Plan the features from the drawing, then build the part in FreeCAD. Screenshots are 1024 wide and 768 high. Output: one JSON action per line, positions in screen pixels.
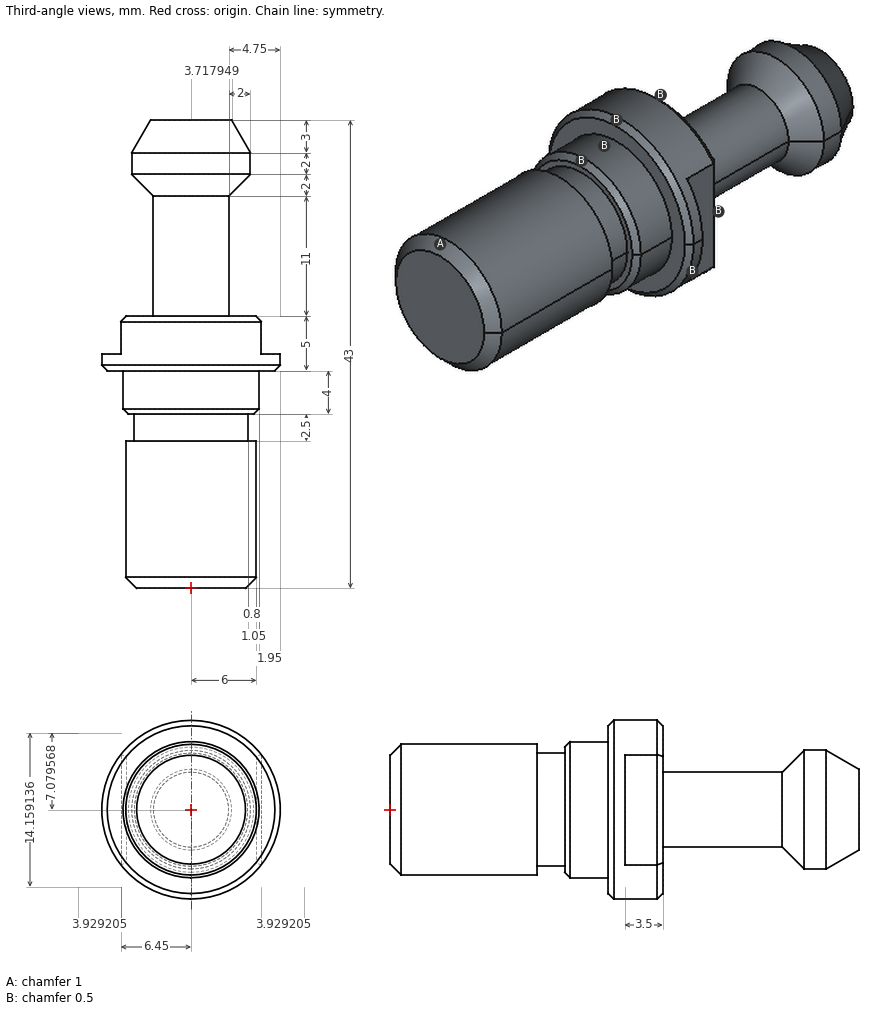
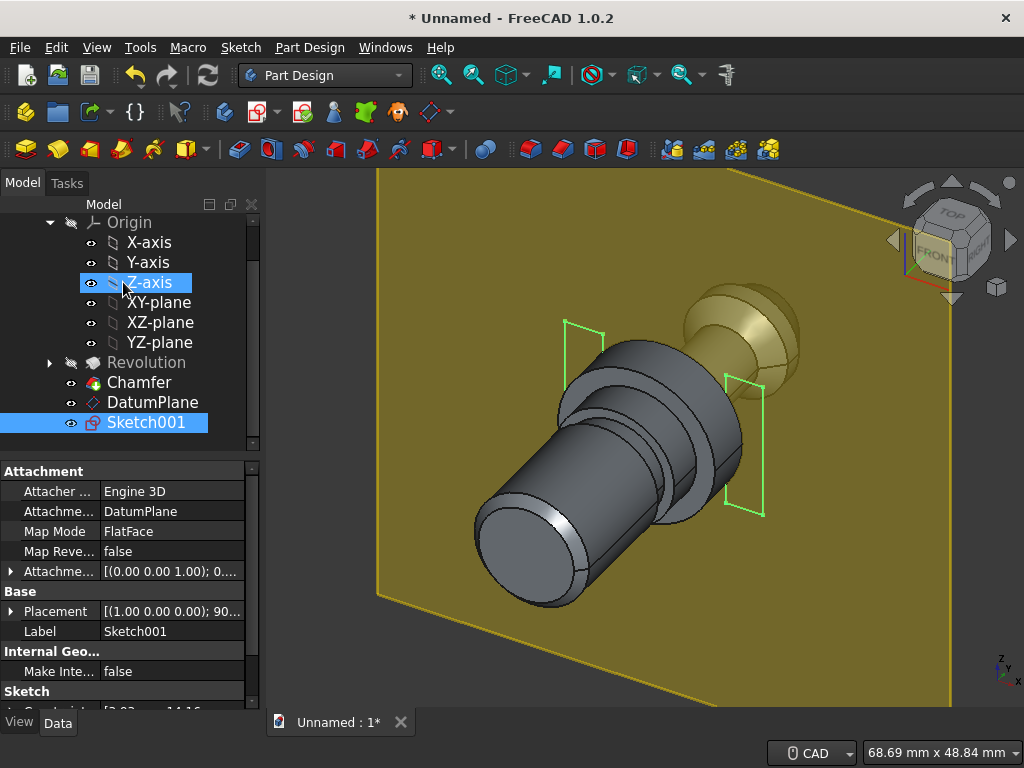
{"action": "left_click", "coordinate": [240, 150]}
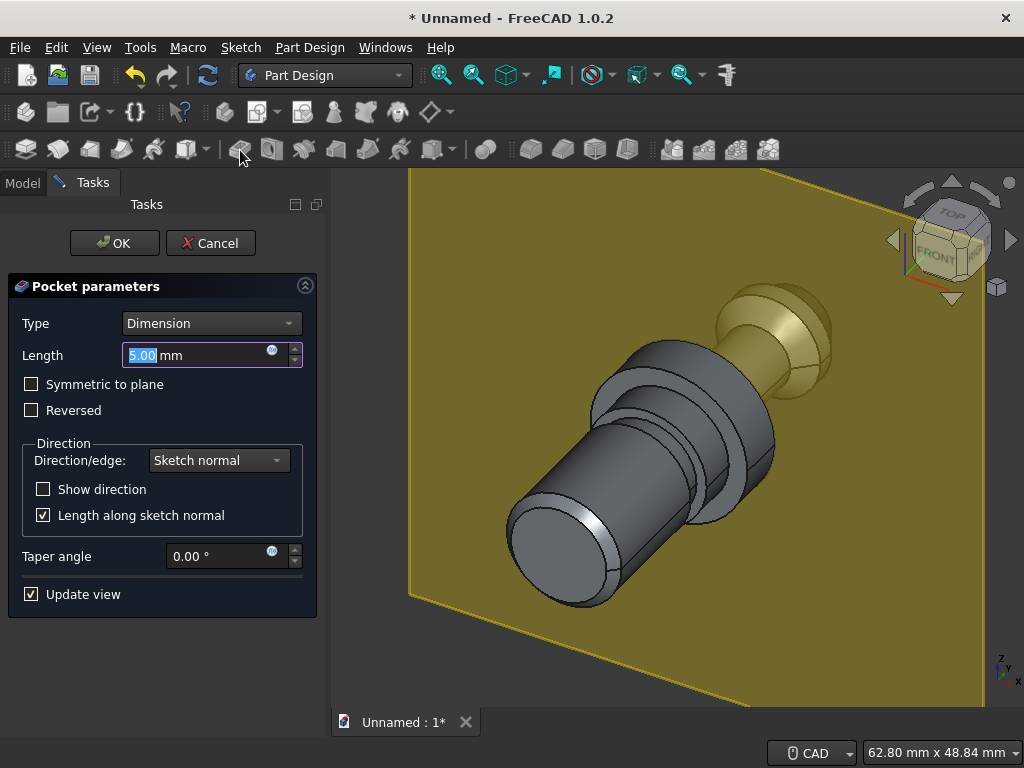
{"action": "type", "text": "3.5"}
{"action": "key", "text": "Tab"}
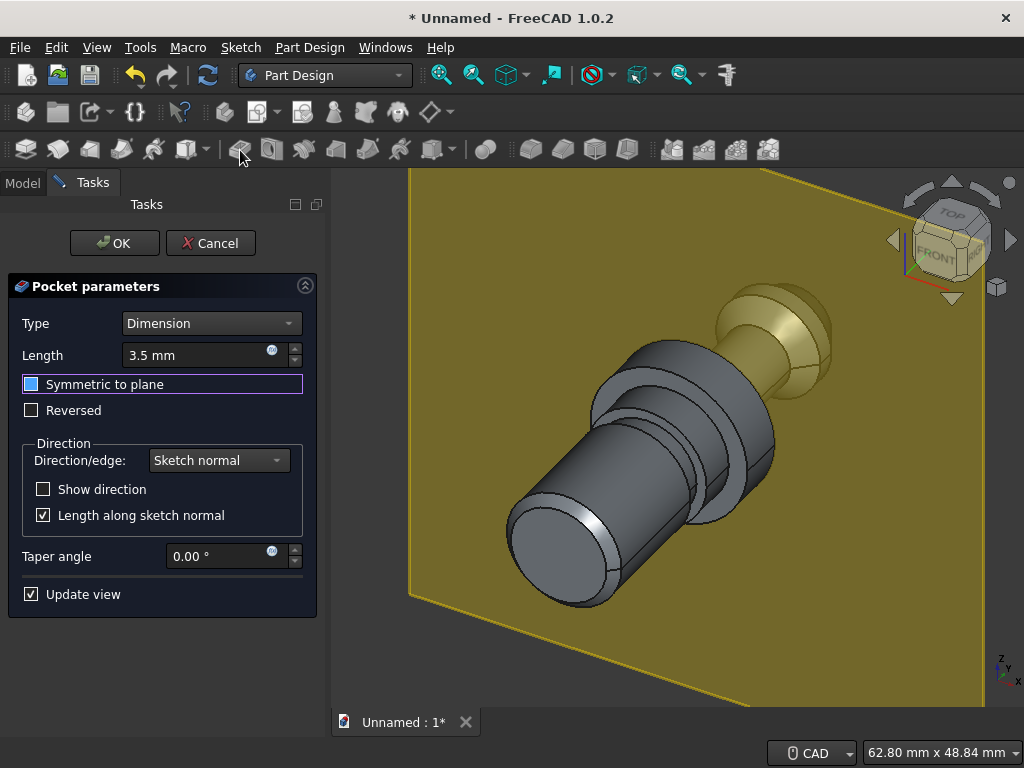
{"action": "left_click", "coordinate": [30, 410]}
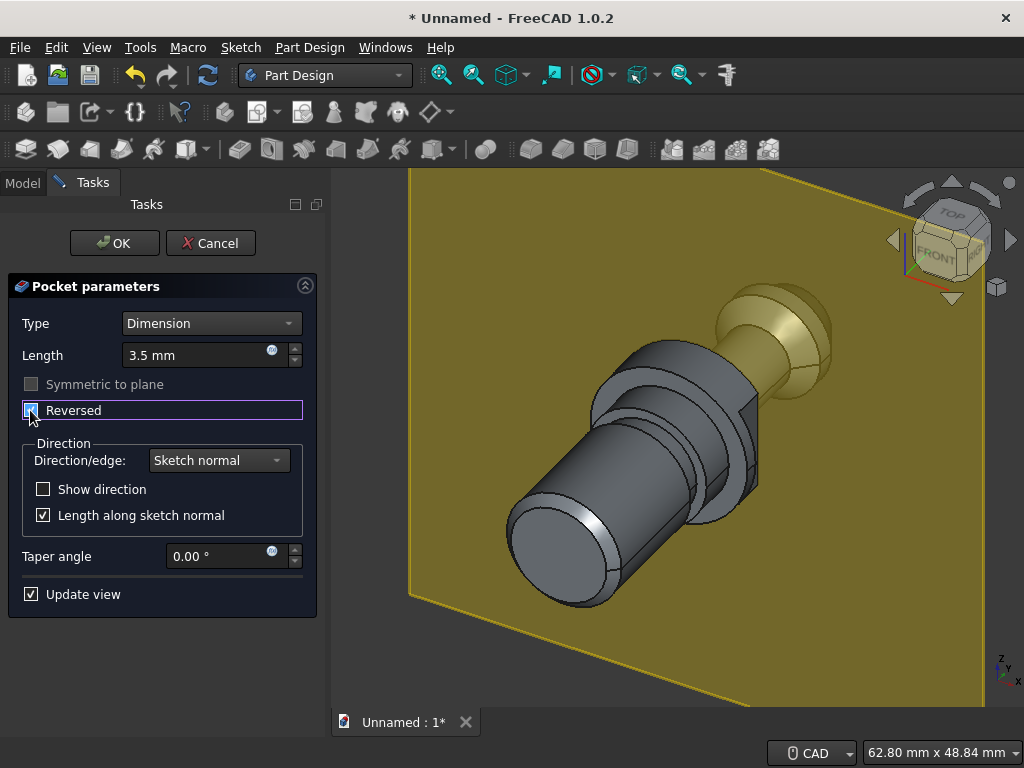
{"action": "left_click", "coordinate": [115, 243]}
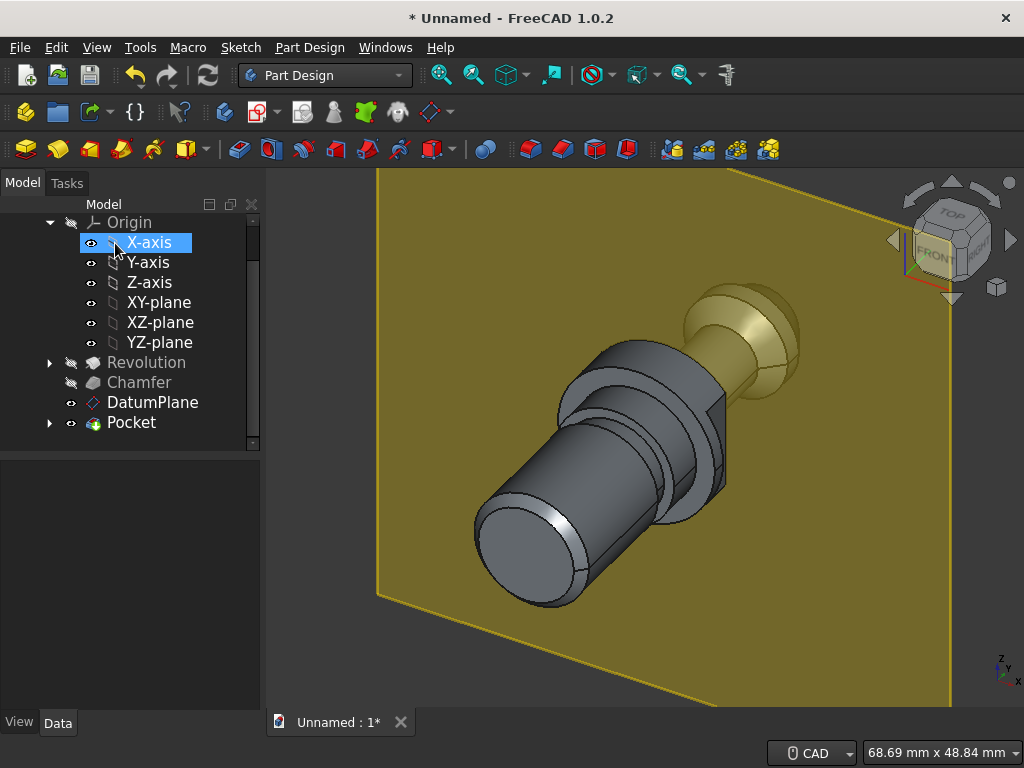
{"action": "left_click", "coordinate": [116, 403]}
{"action": "key", "text": "space"}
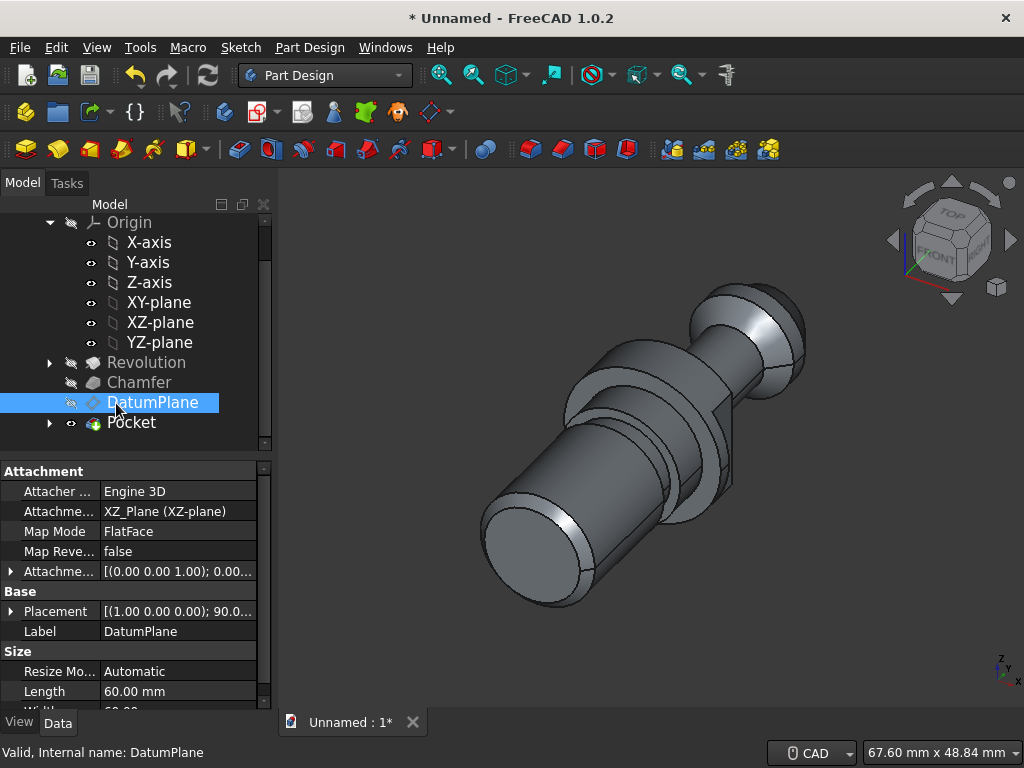
{"action": "left_click", "coordinate": [572, 417]}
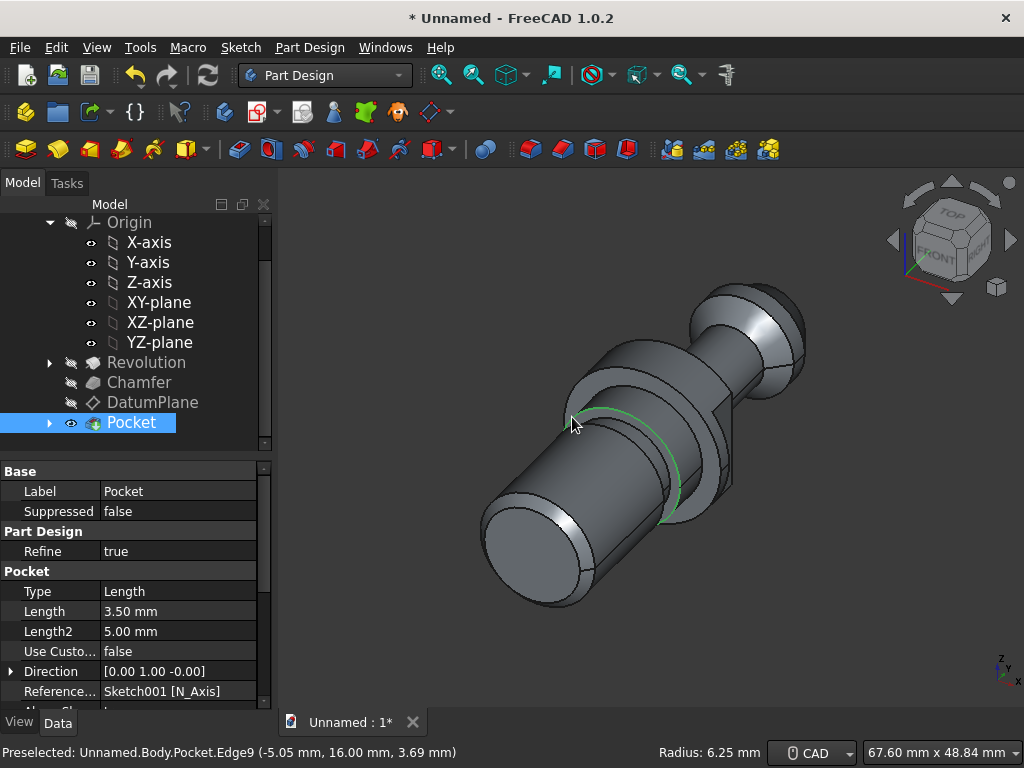
{"action": "left_click", "coordinate": [618, 366], "text": "ctrl"}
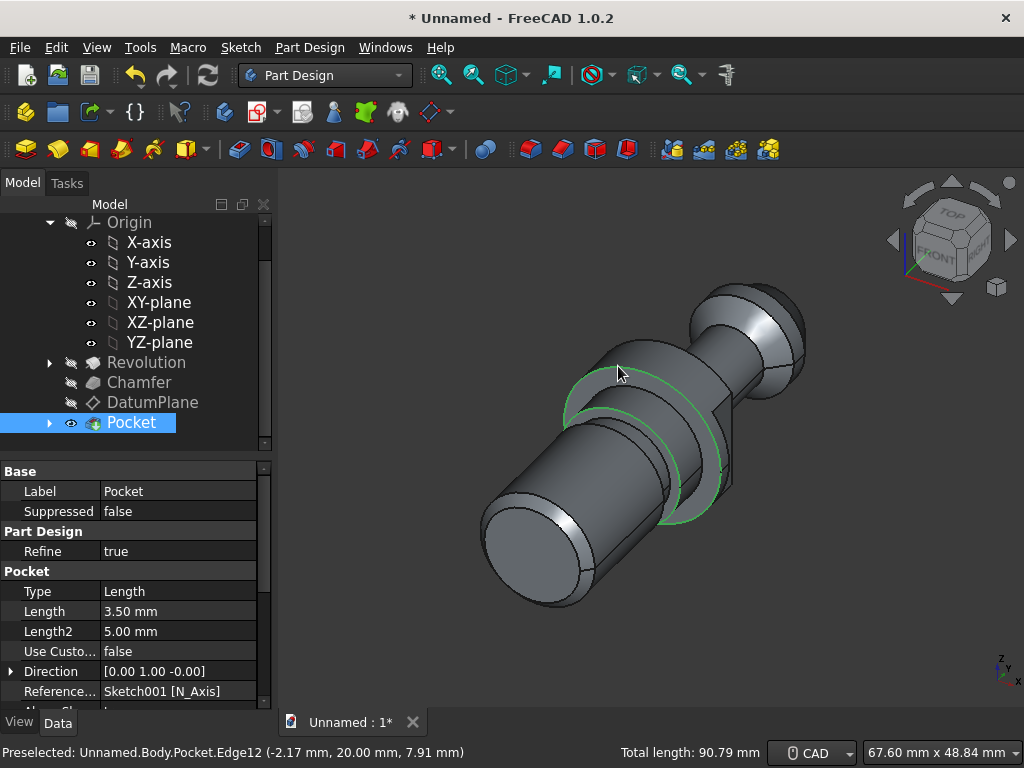
{"action": "key", "text": "0"}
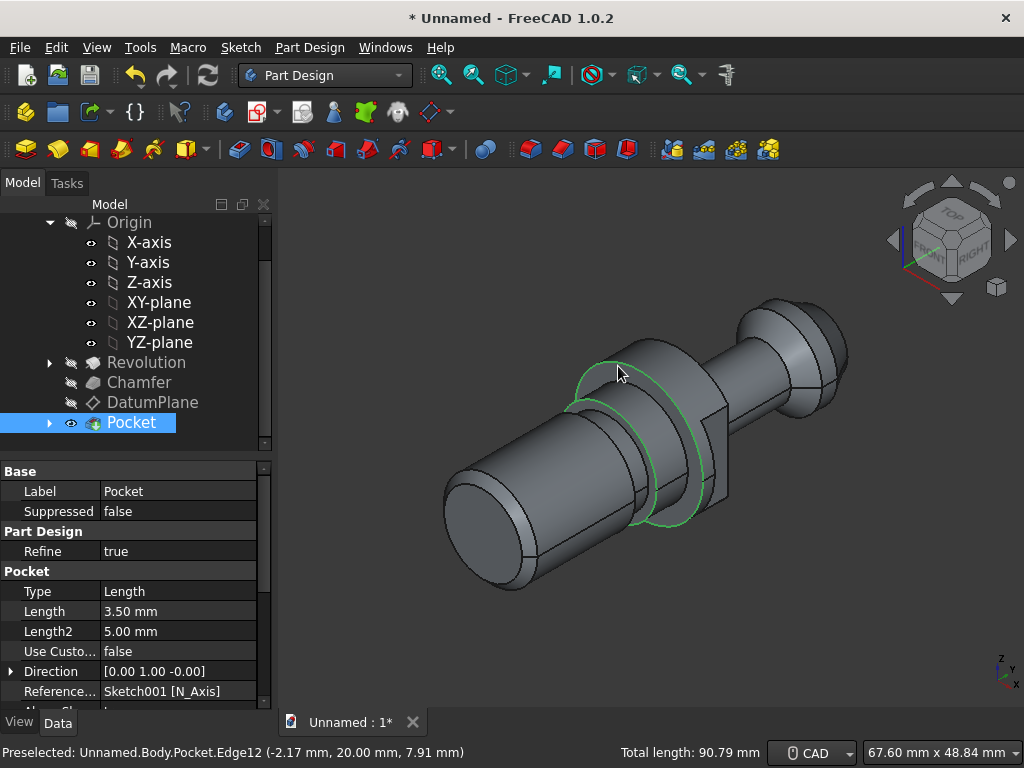
{"action": "left_click", "coordinate": [667, 341], "text": "ctrl"}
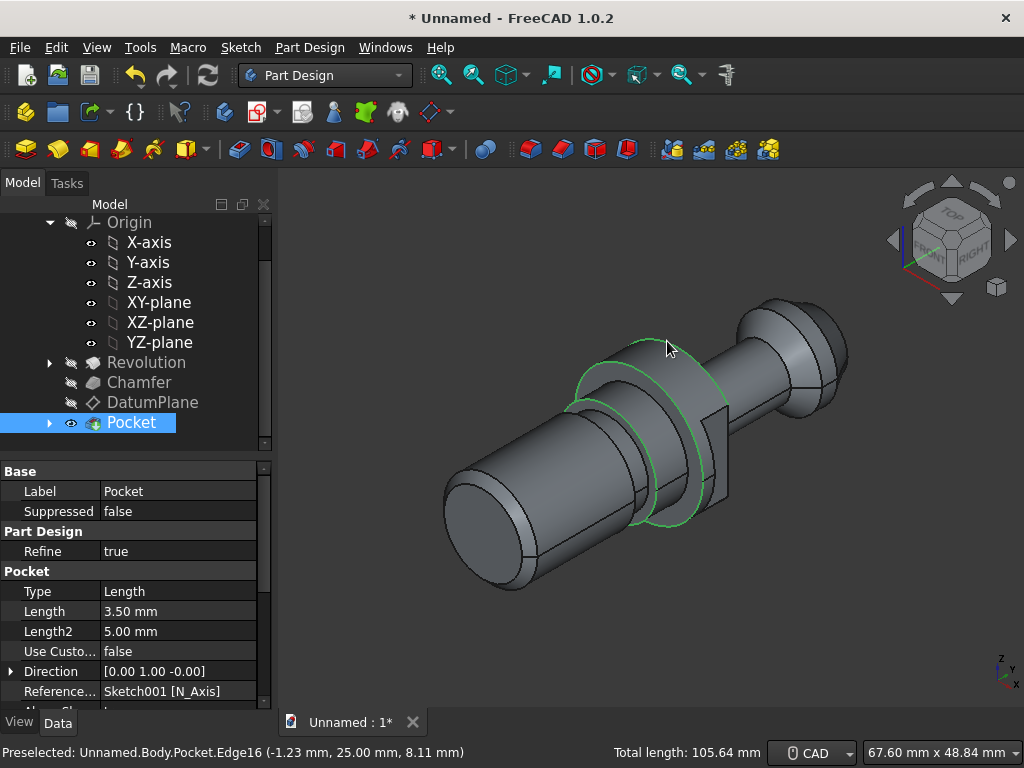
{"action": "key", "text": "2"}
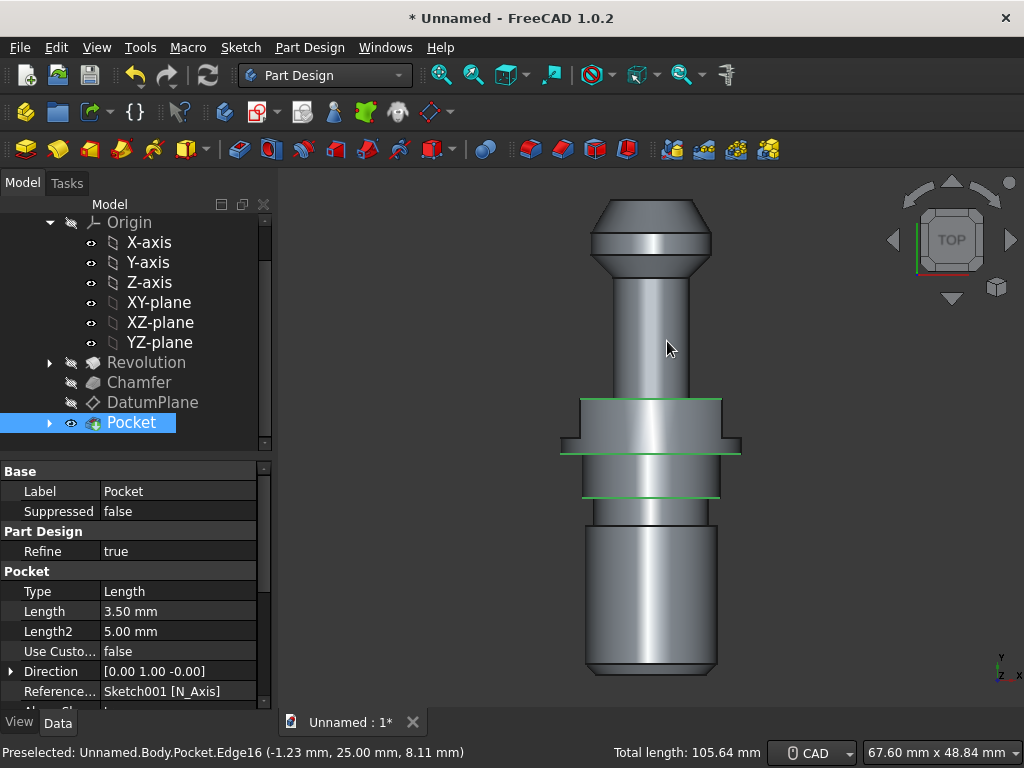
{"action": "key", "text": "1"}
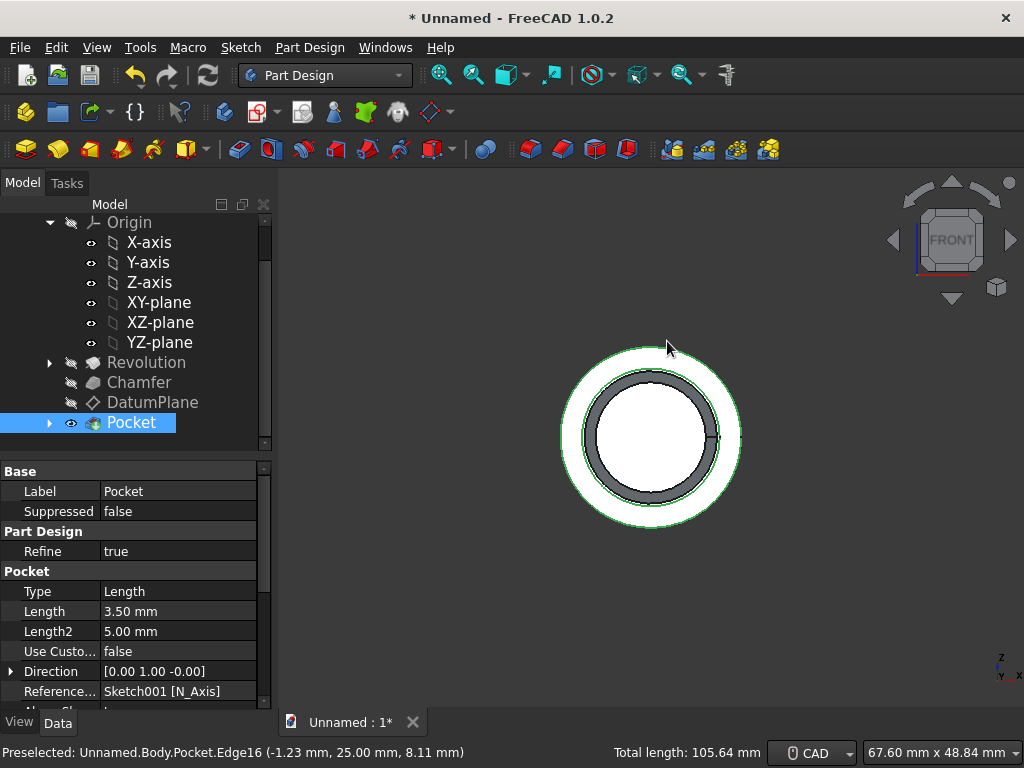
{"action": "left_click", "coordinate": [442, 76]}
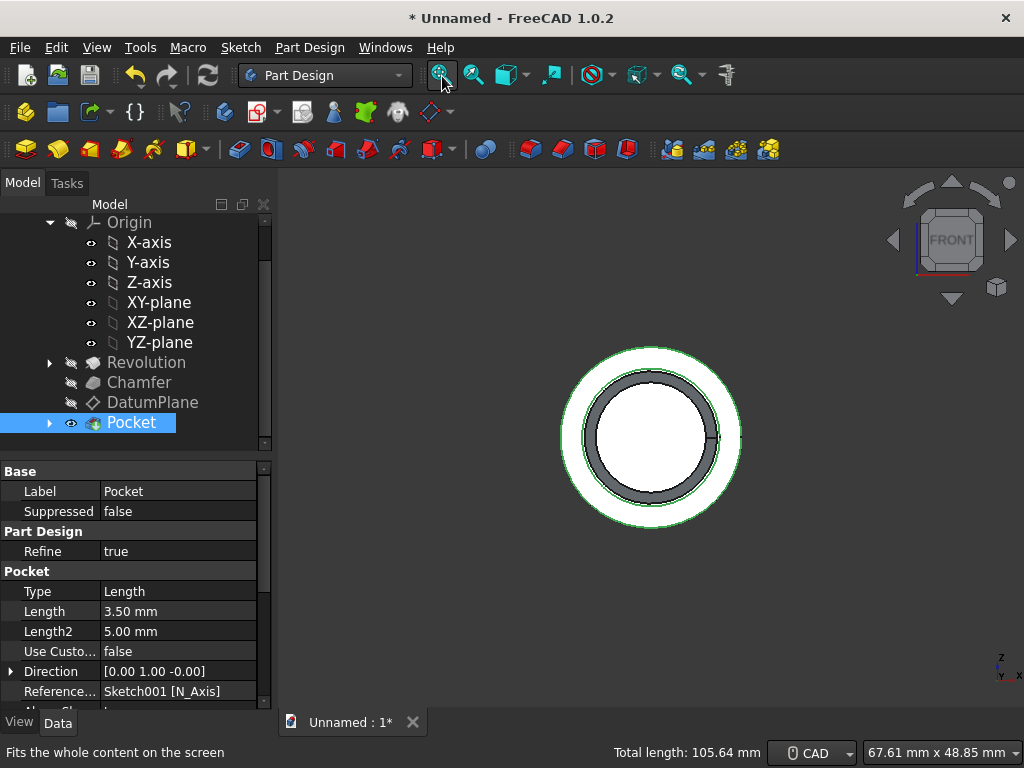
{"action": "key", "text": "3"}